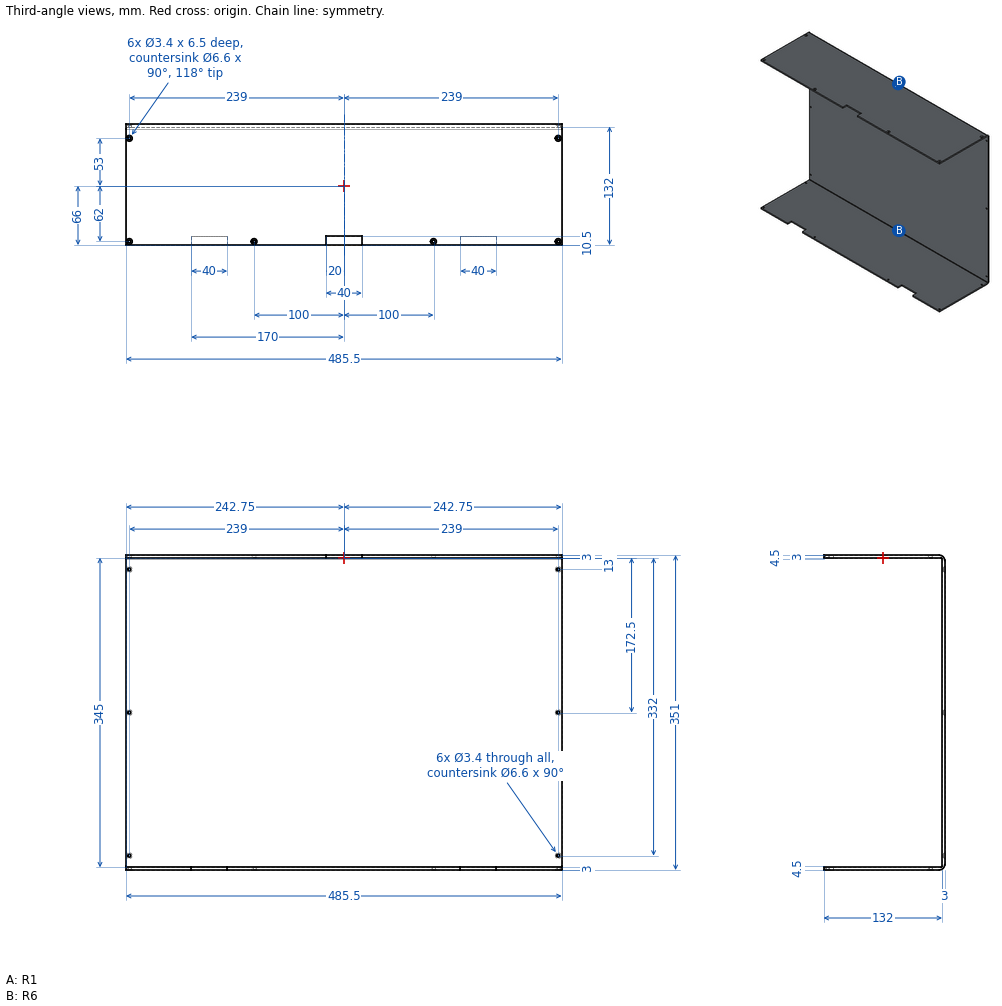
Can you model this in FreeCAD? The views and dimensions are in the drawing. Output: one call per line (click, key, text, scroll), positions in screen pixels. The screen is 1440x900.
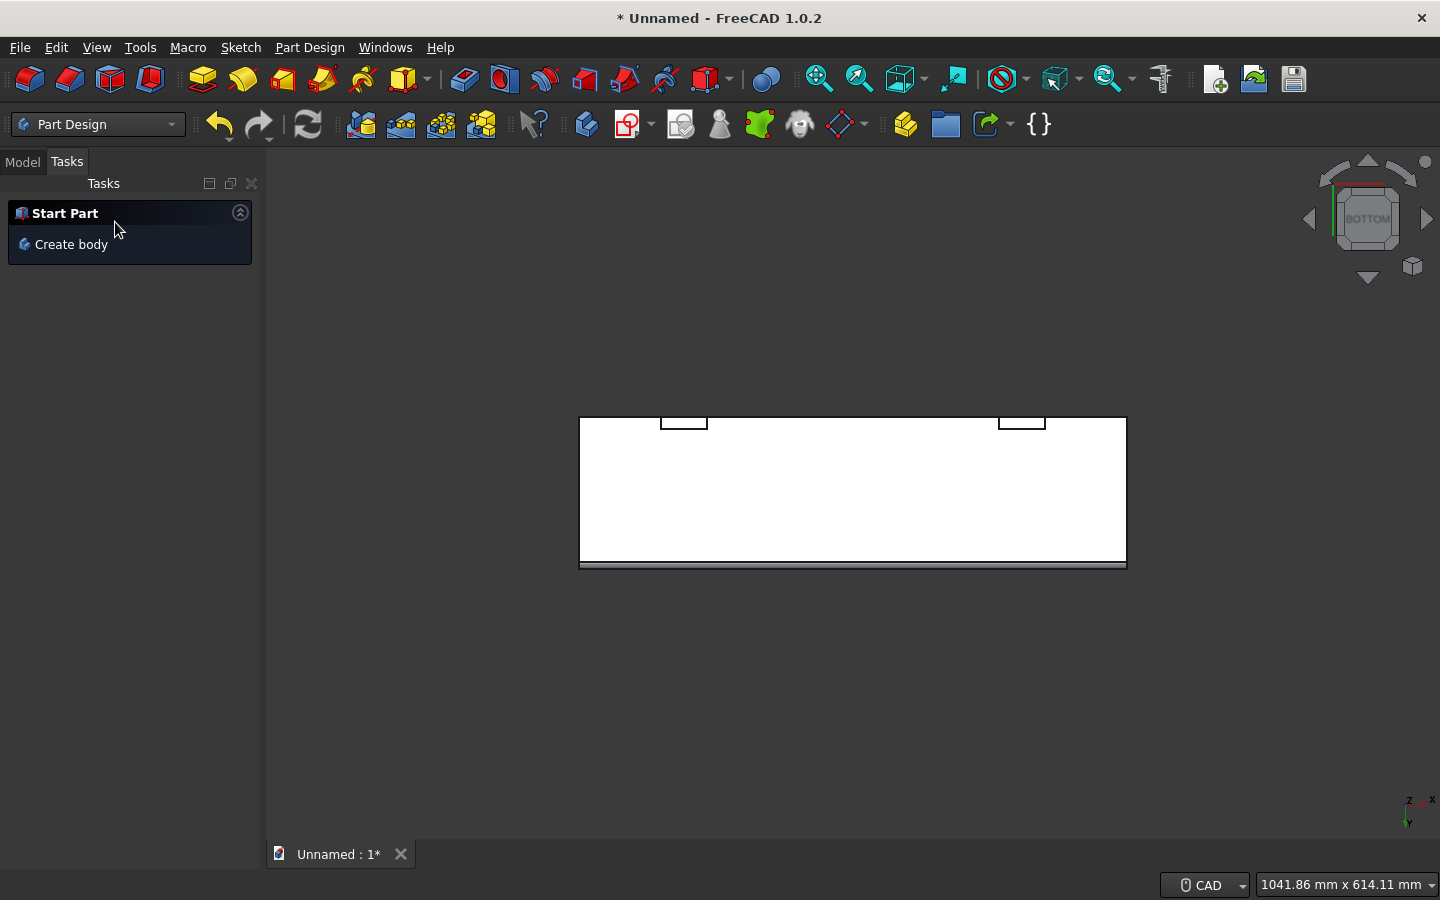
key(4)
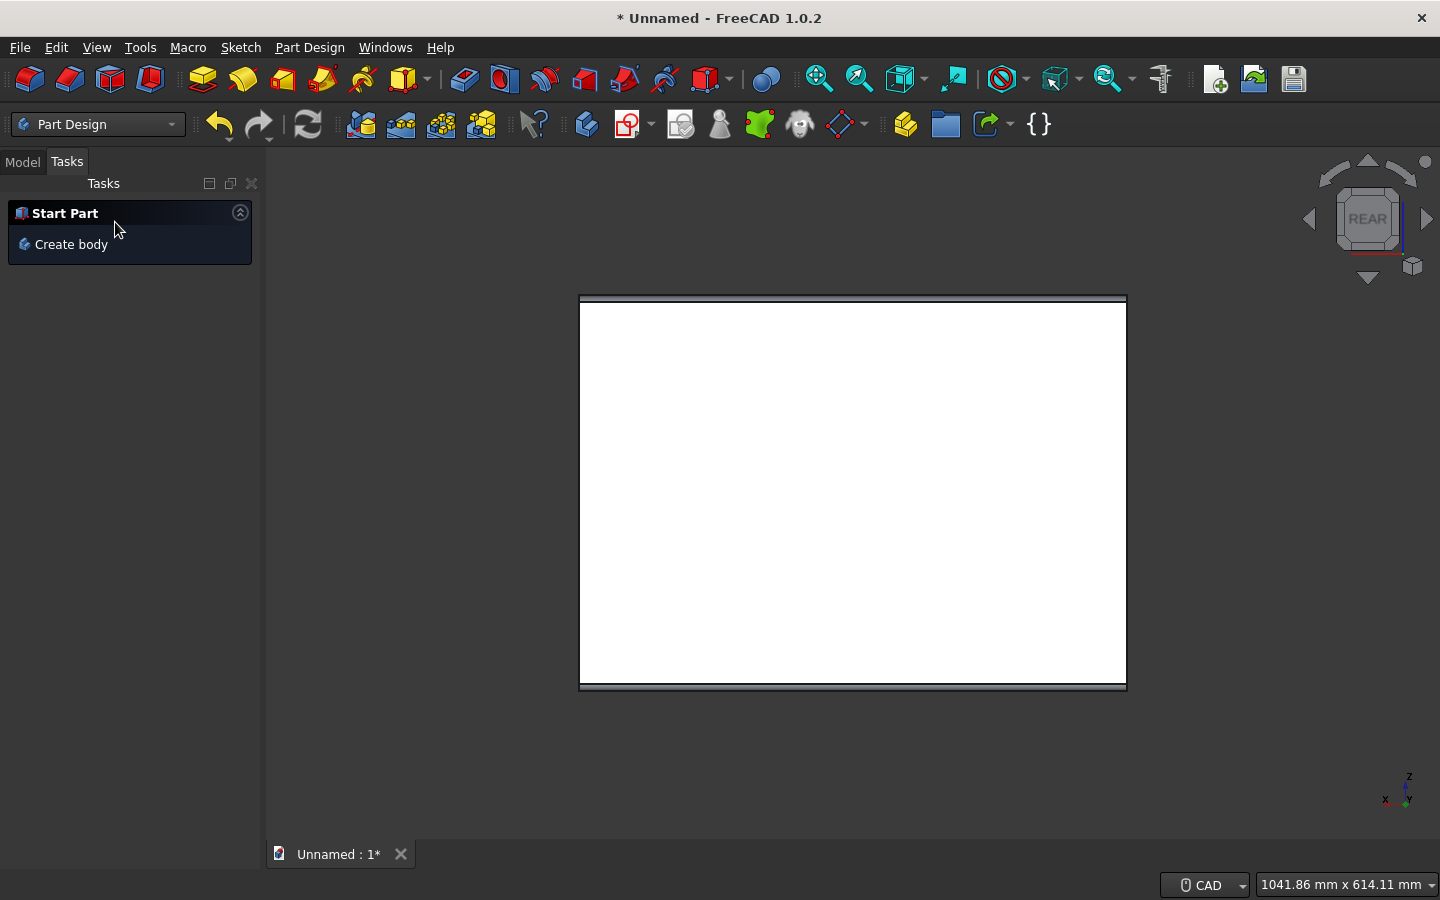
click(775, 492)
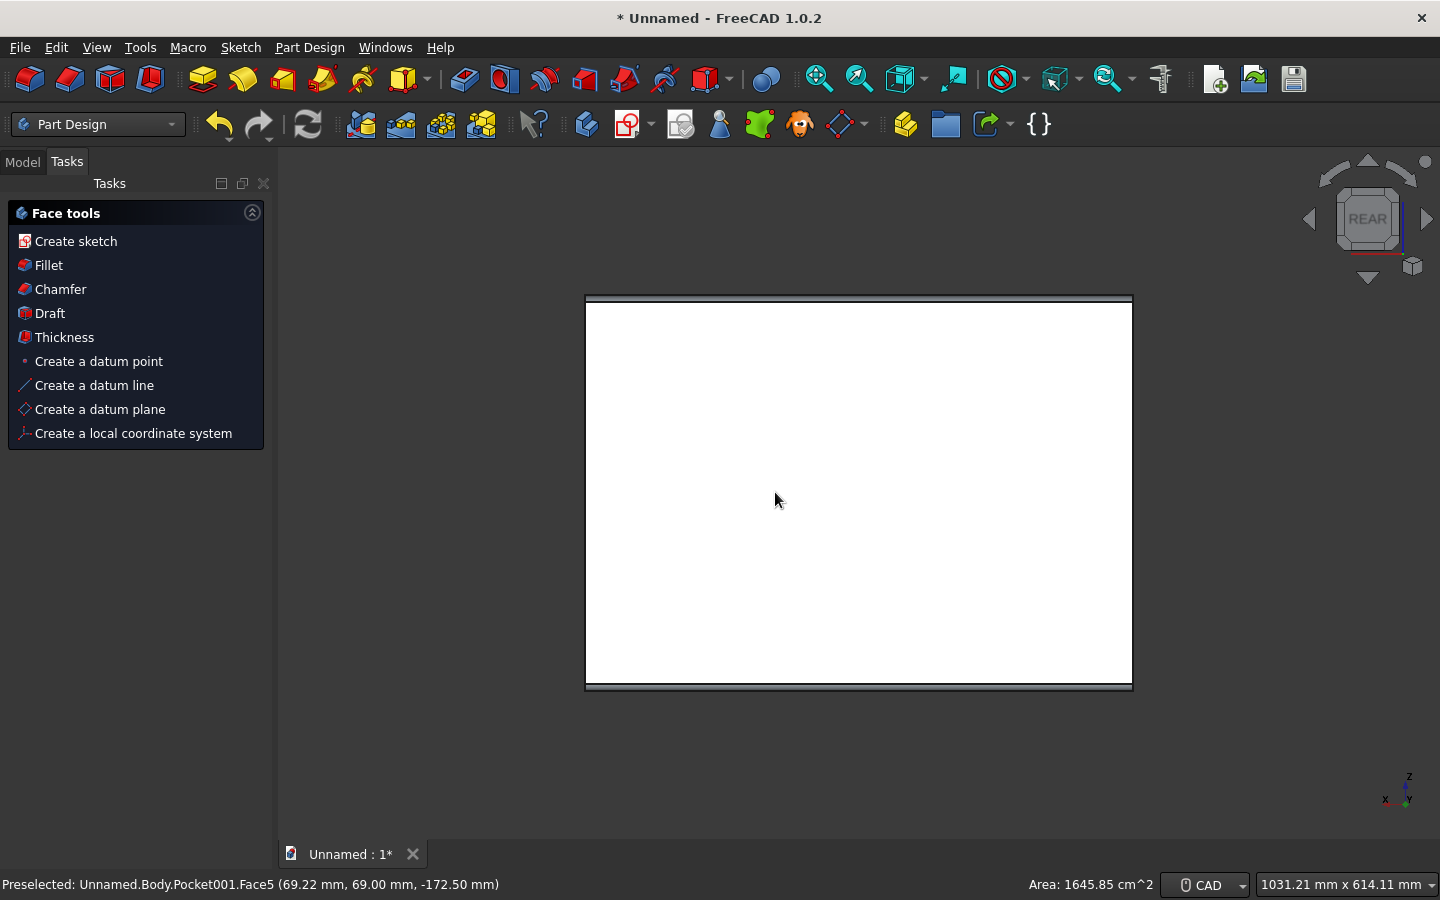
click(628, 124)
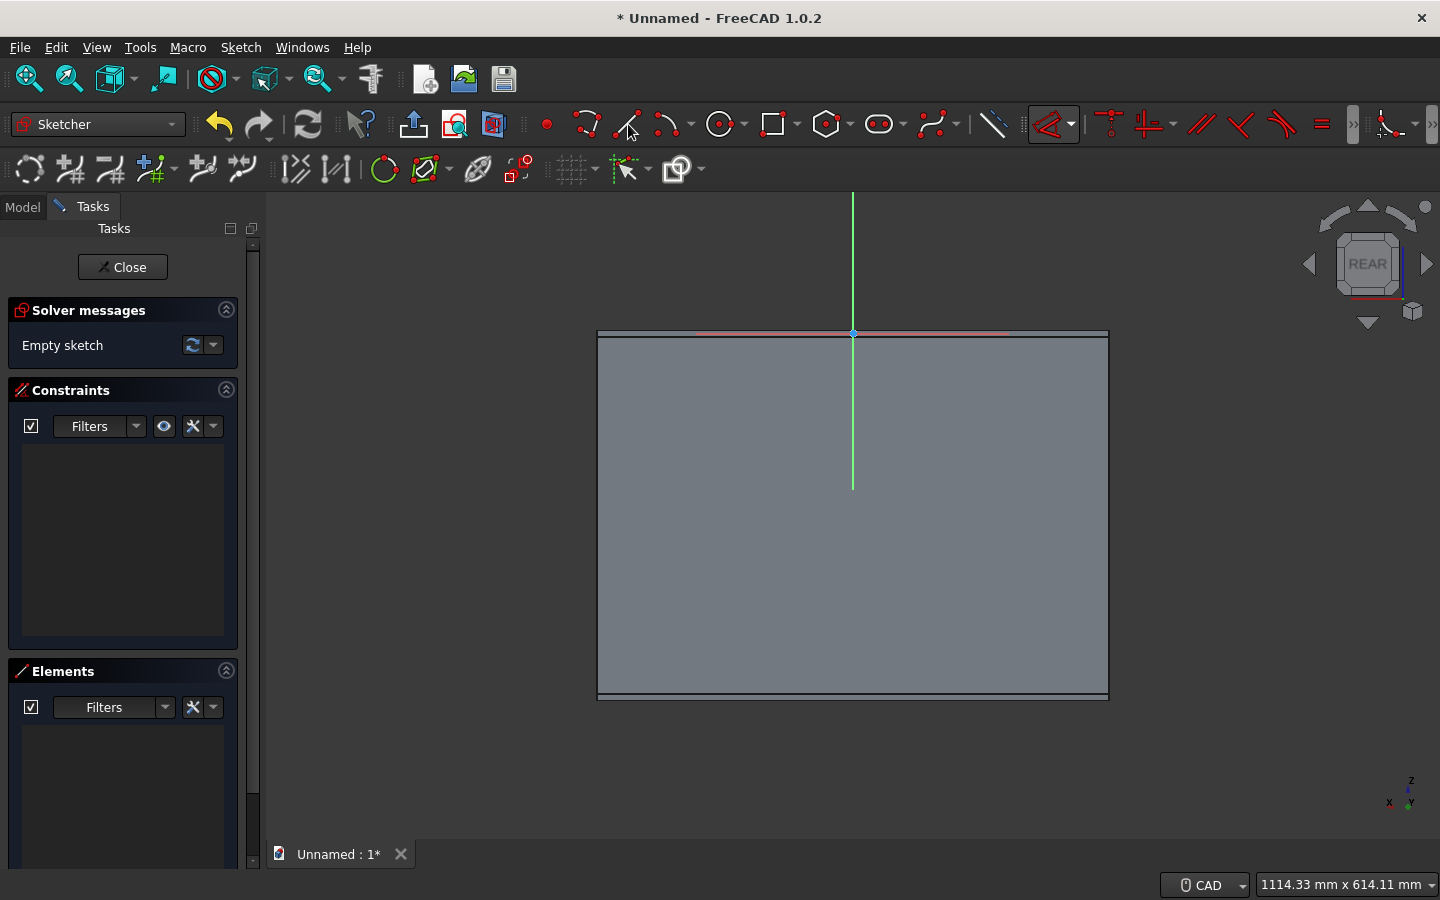
click(720, 124)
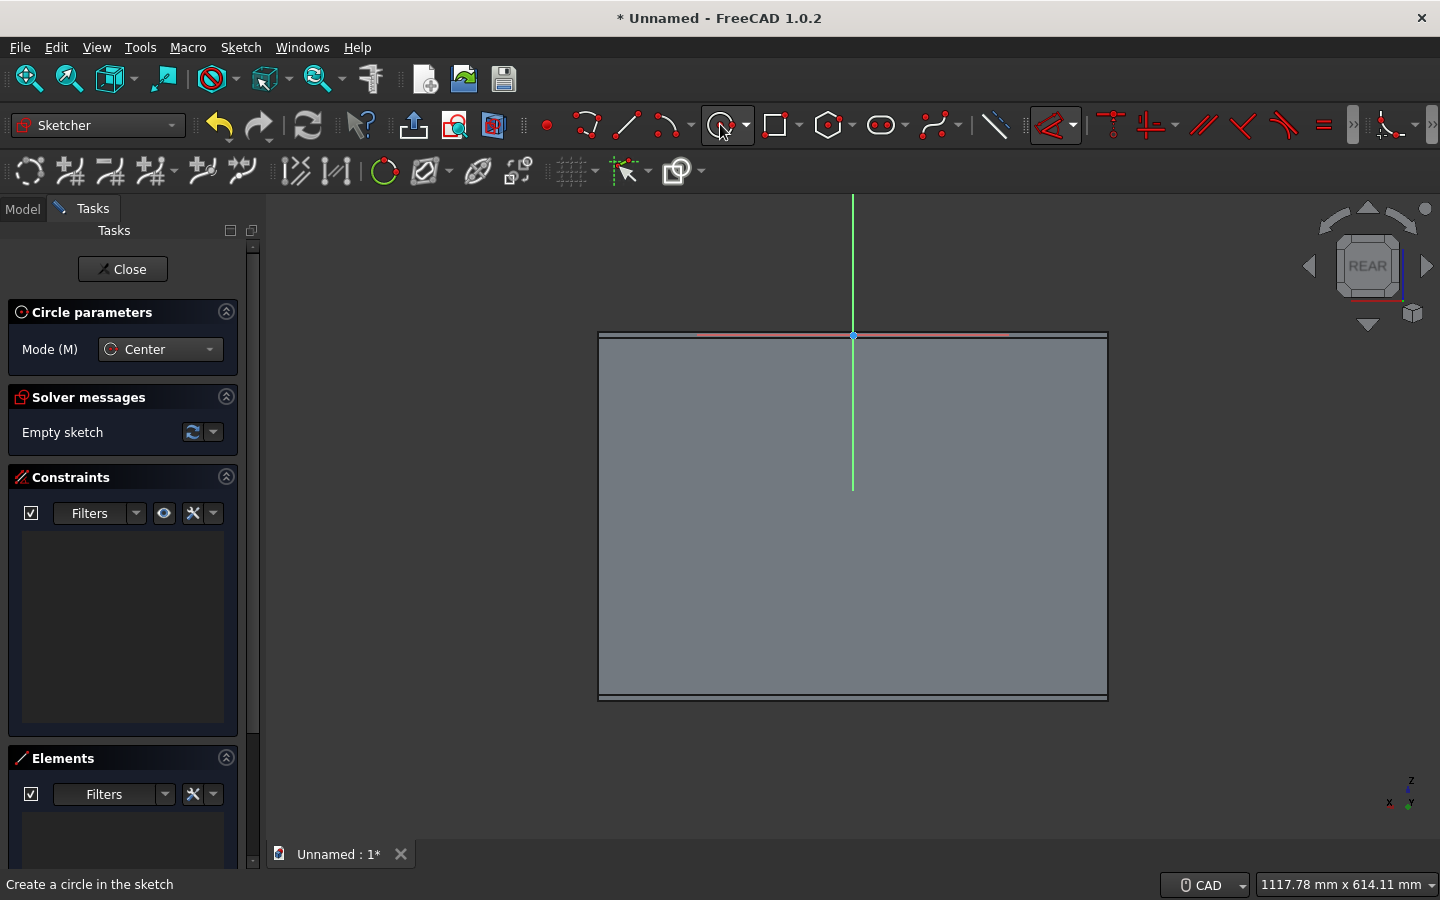
scroll(602, 684, up, 13)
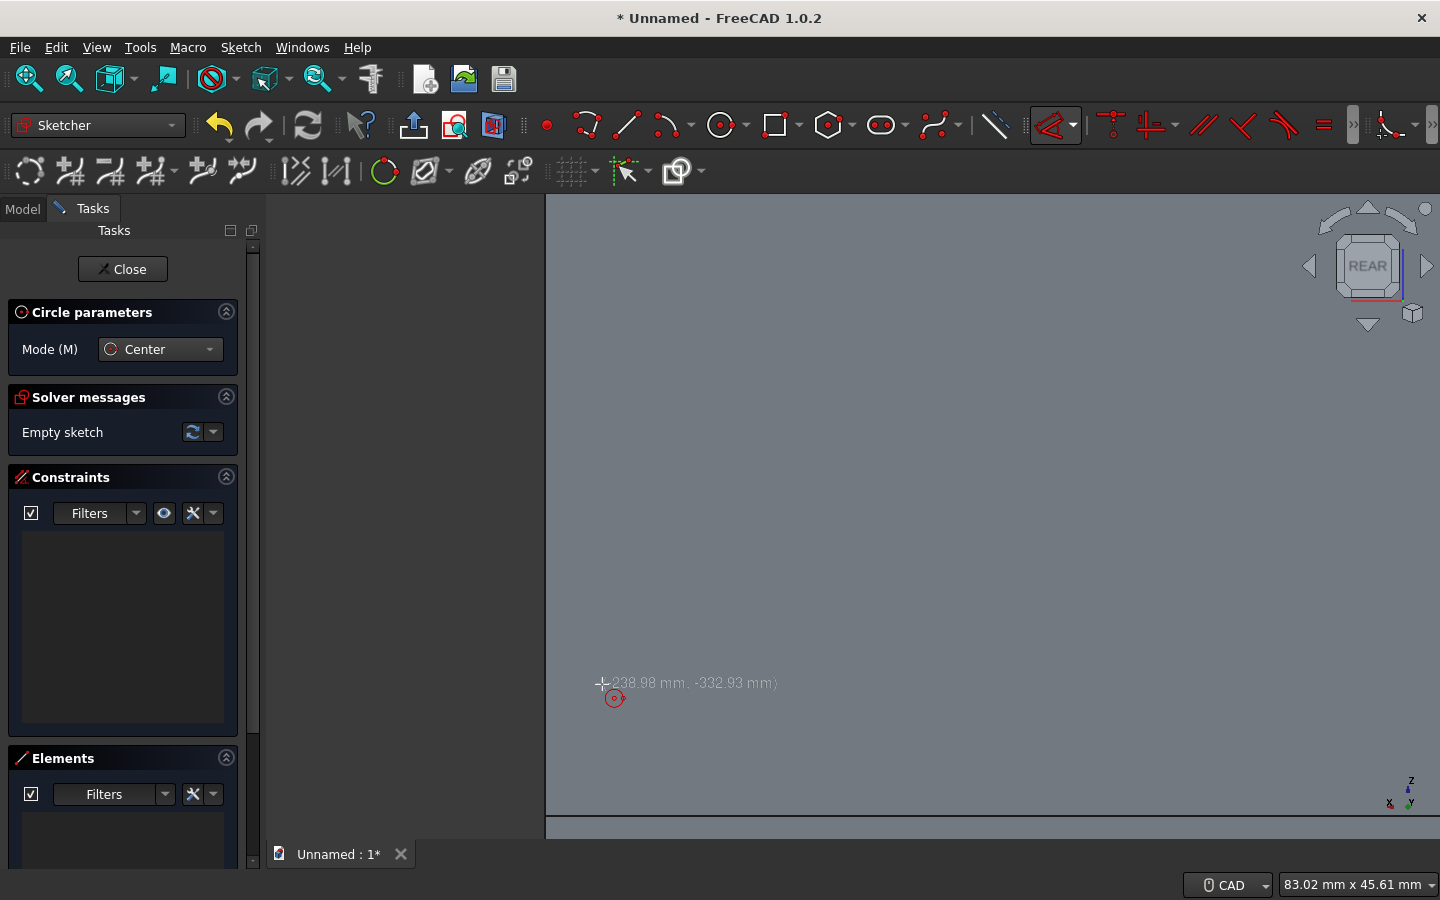
scroll(466, 734, down, 12)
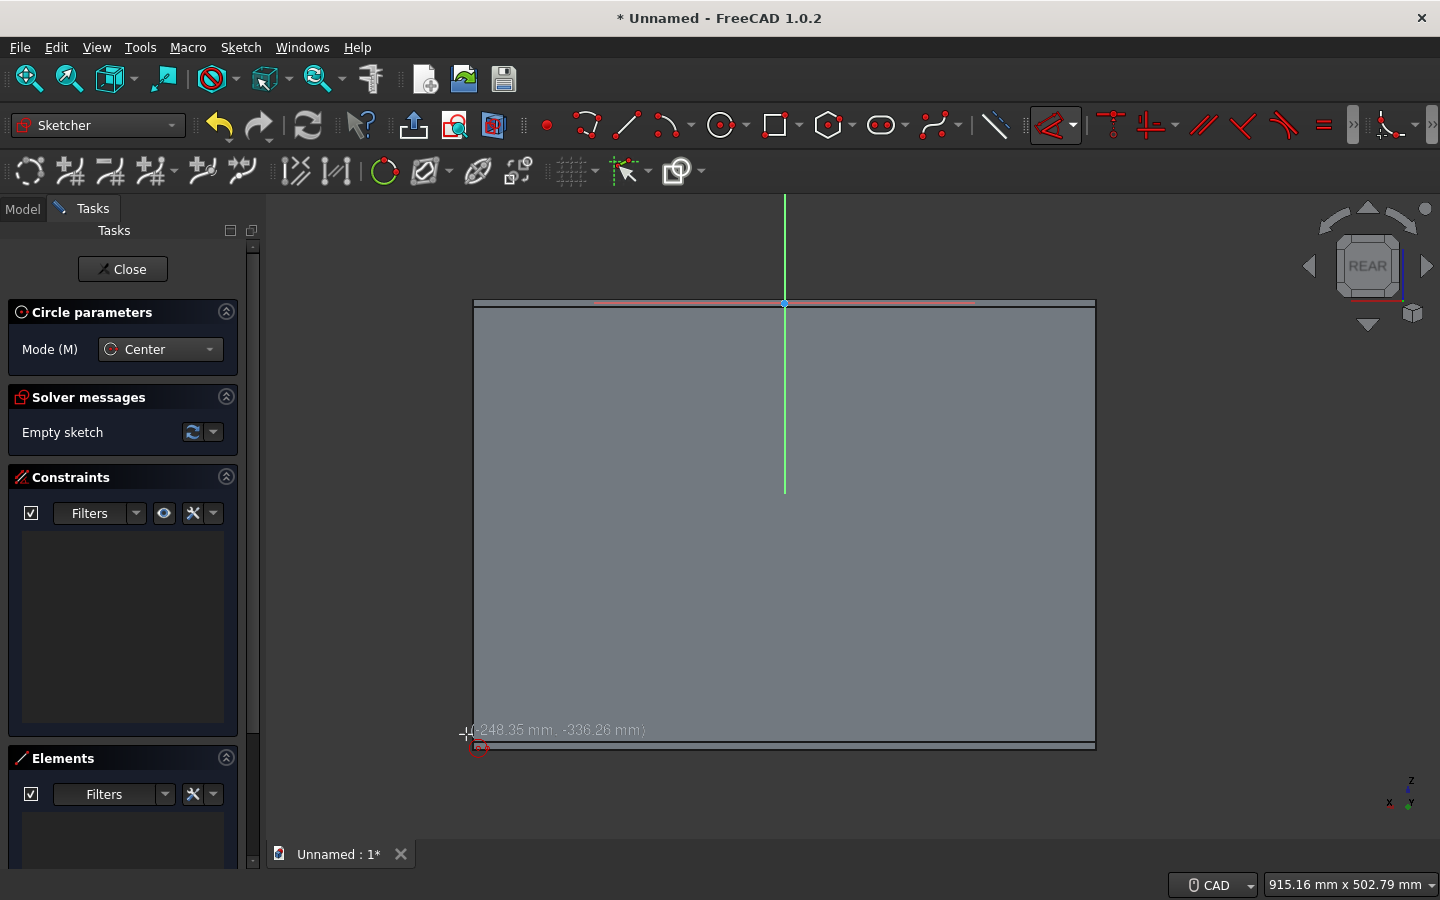
click(478, 729)
move(480, 728)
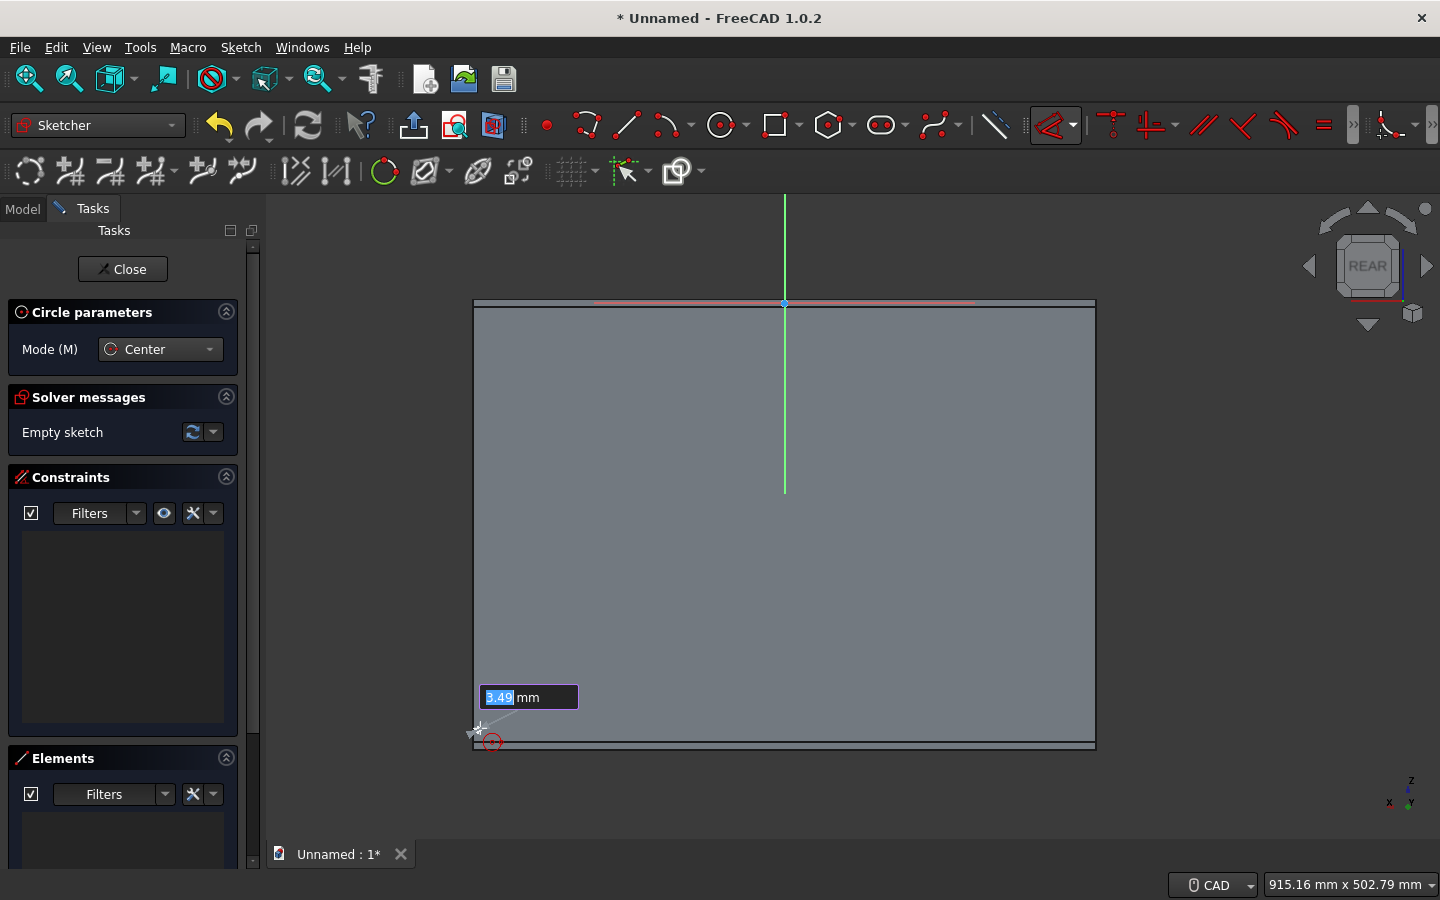
text(3.4)
key(Return)